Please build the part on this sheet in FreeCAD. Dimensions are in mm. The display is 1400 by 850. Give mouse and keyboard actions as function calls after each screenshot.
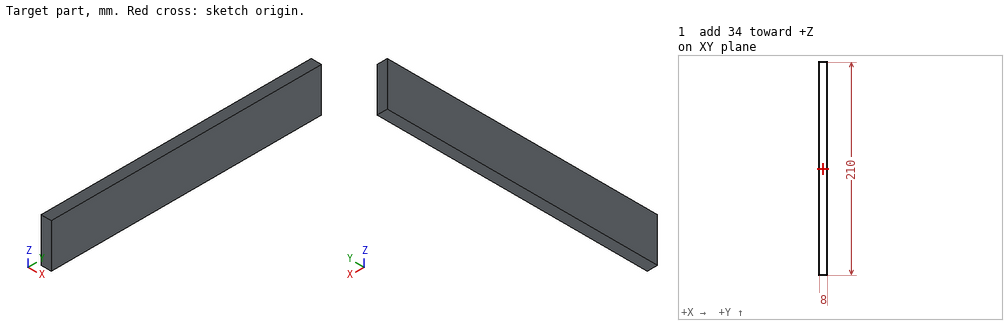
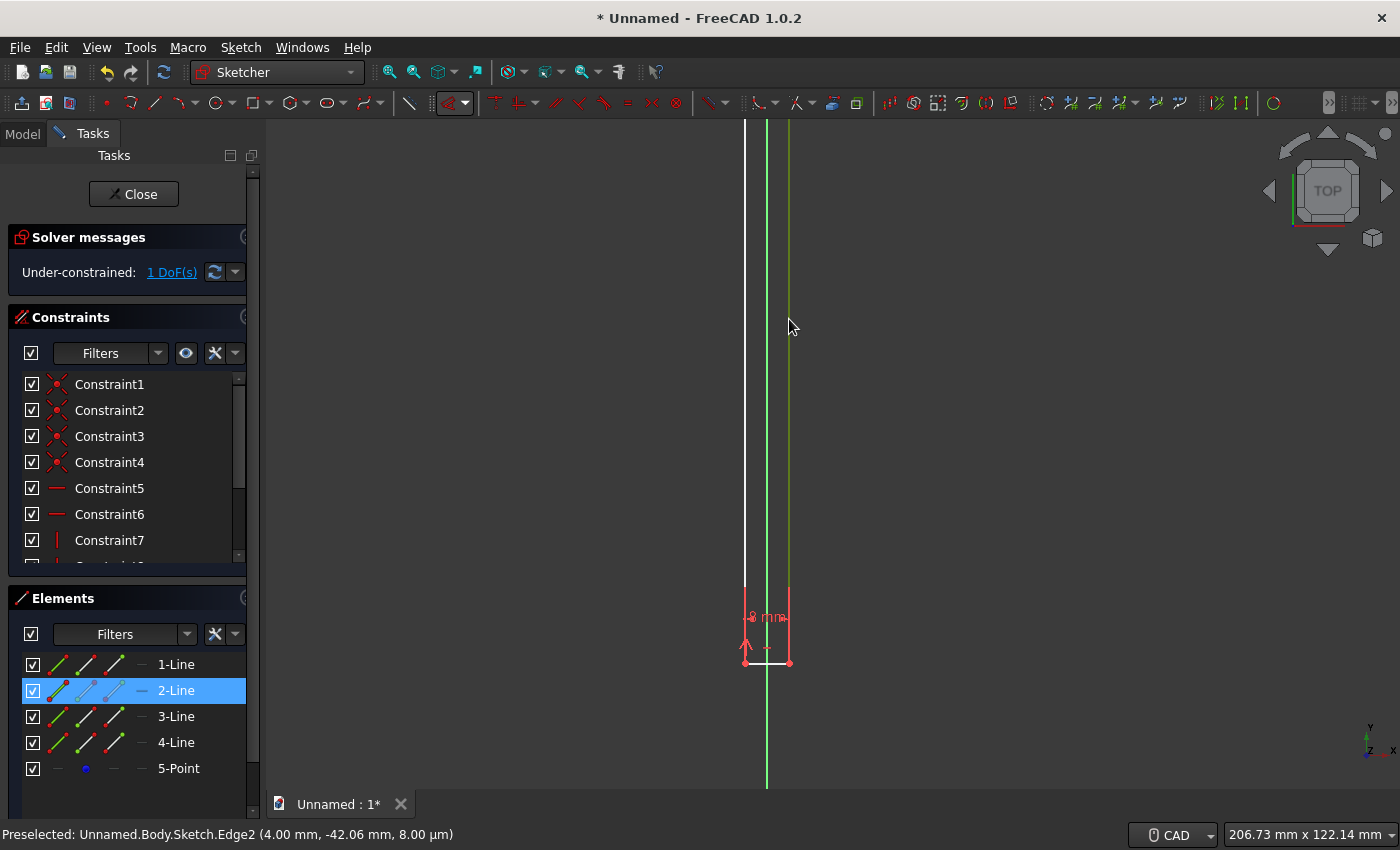
key(i)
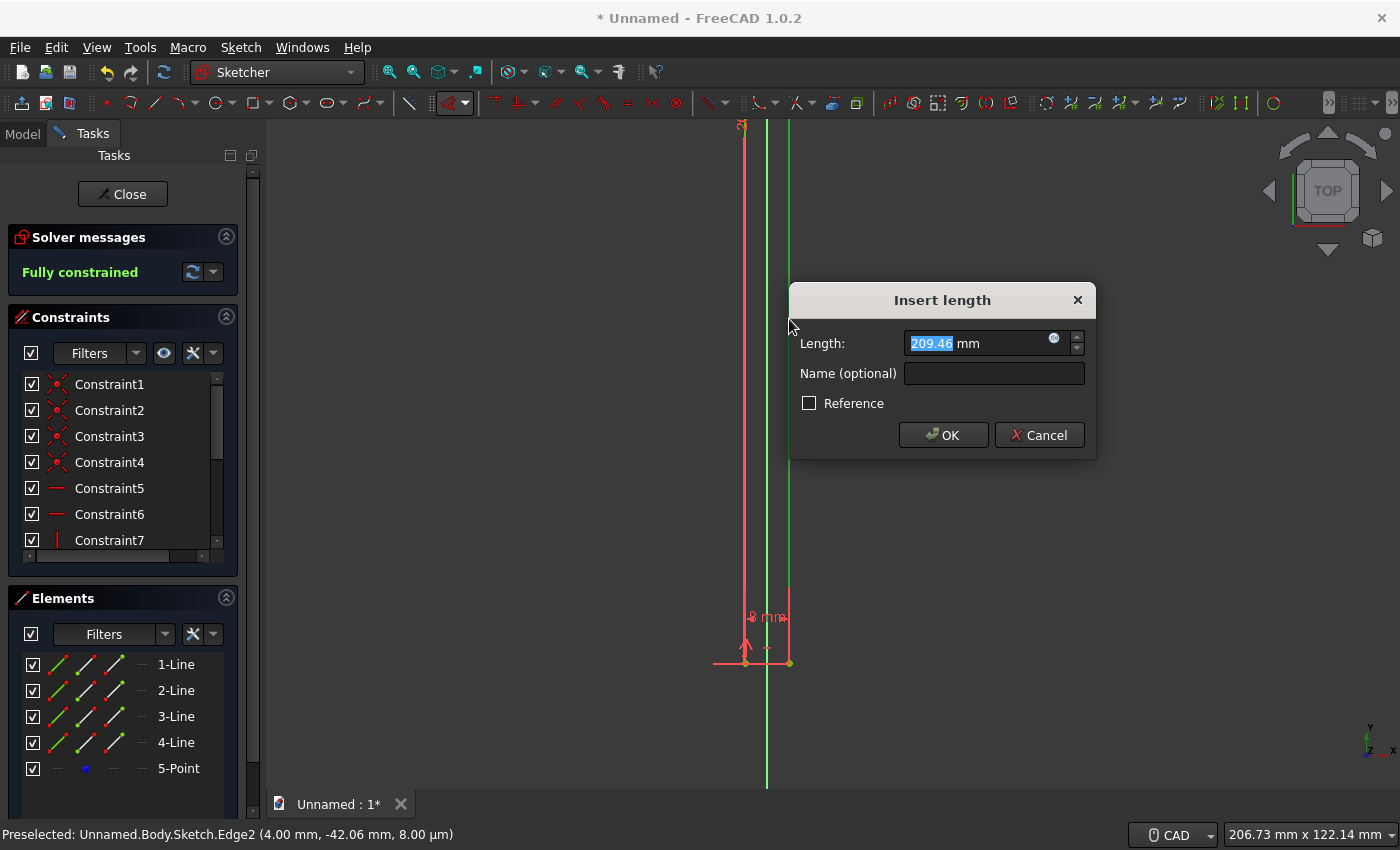
text(210)
key(Return)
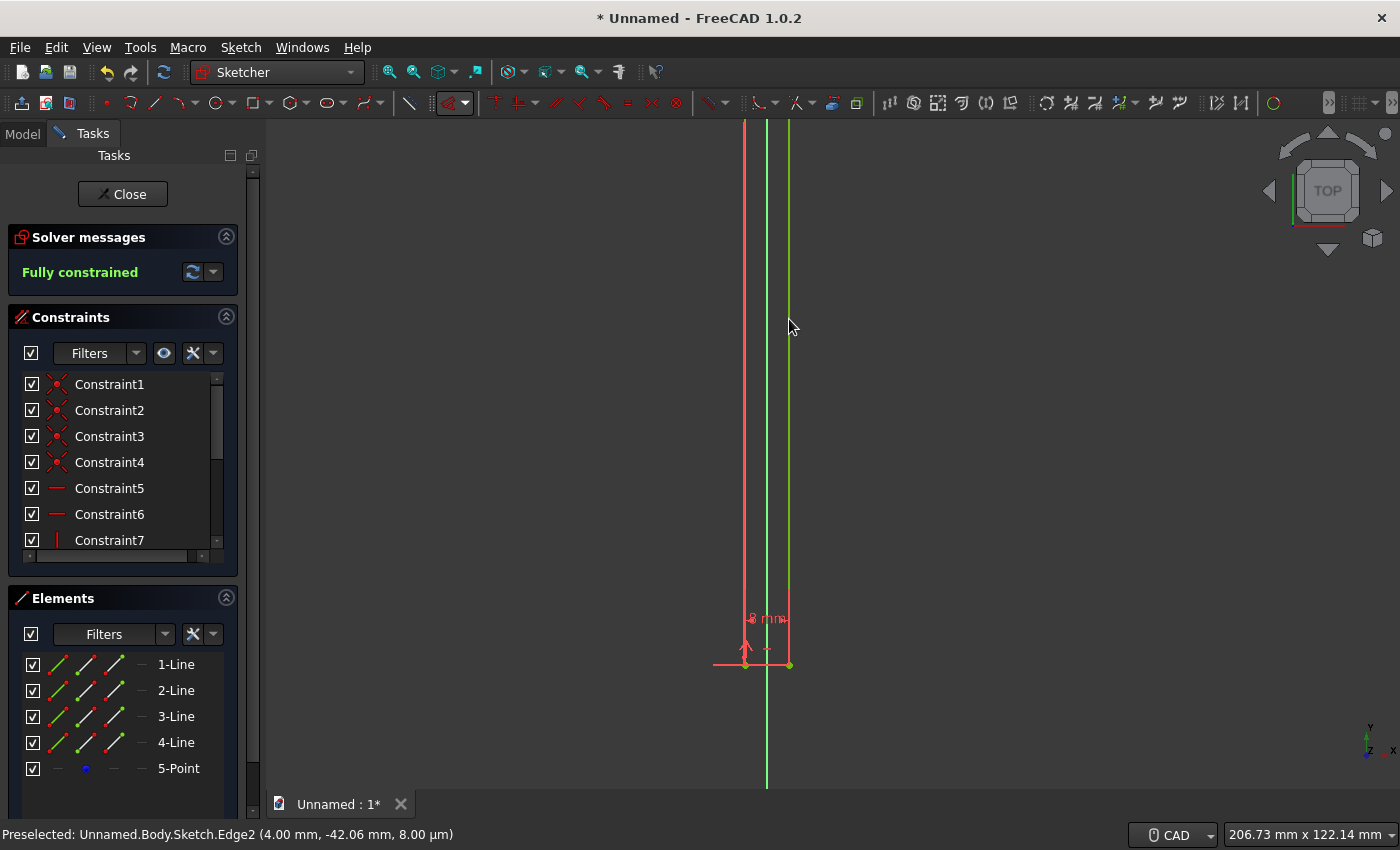
click(123, 194)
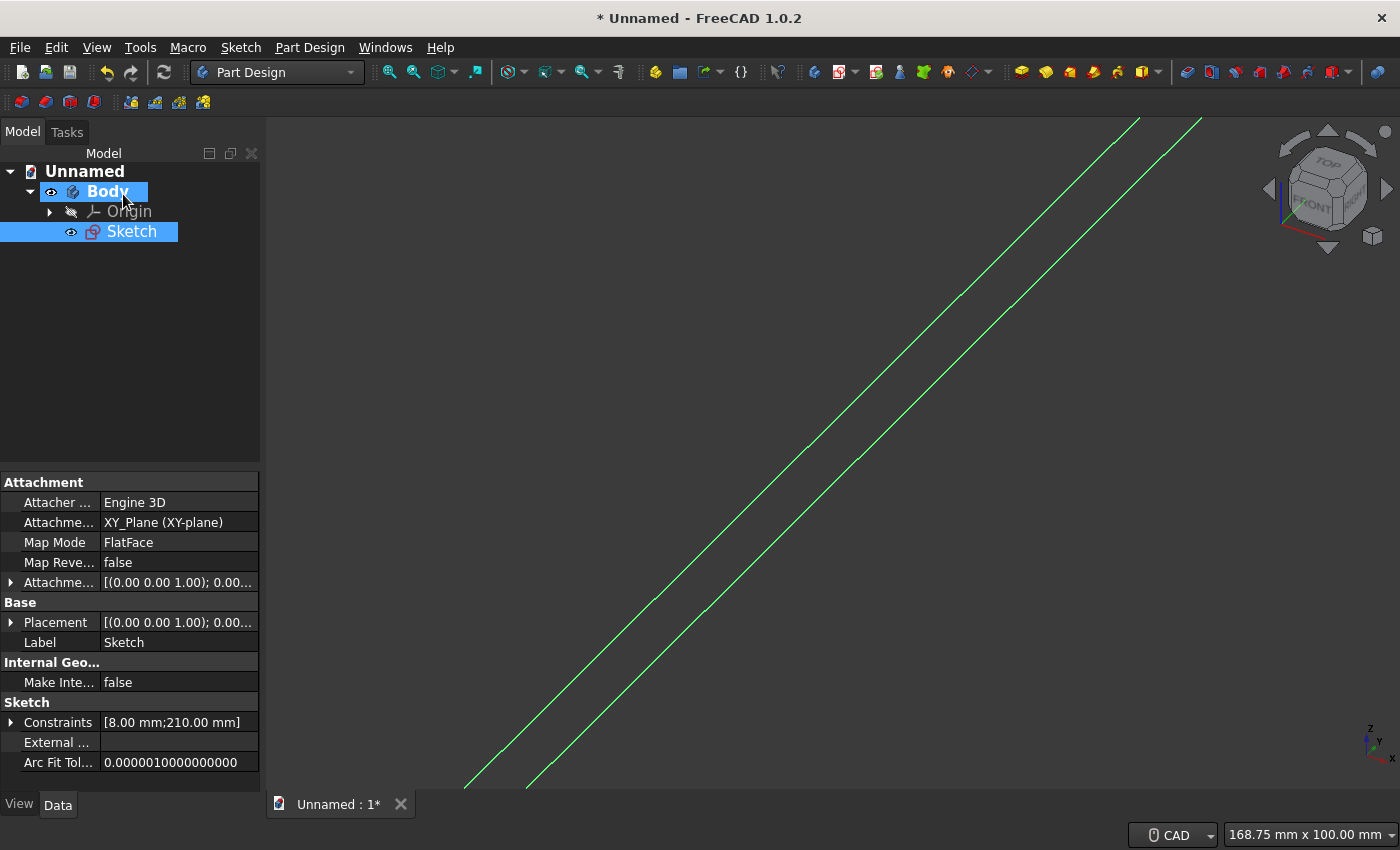
click(1022, 72)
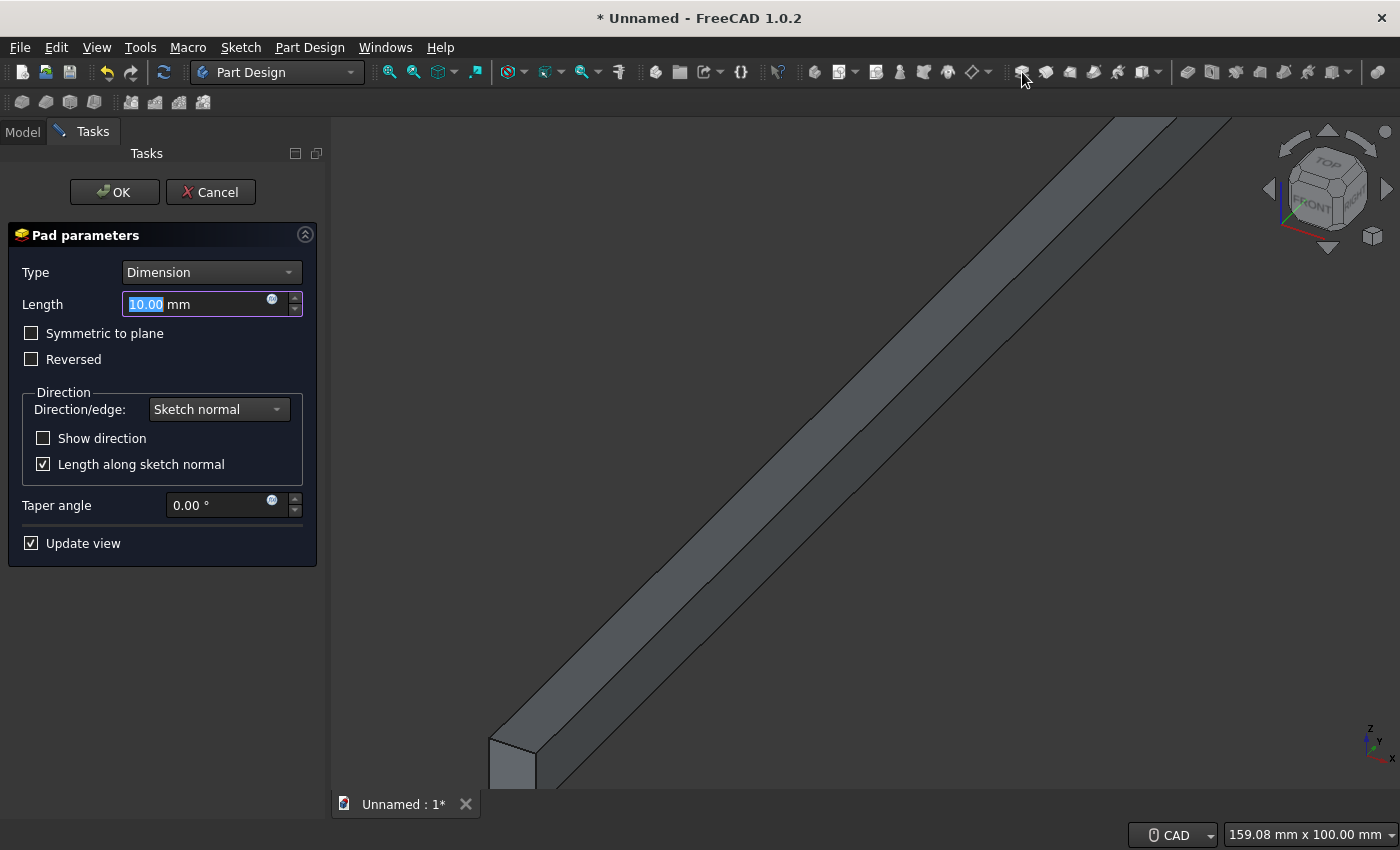
text(34)
key(Tab)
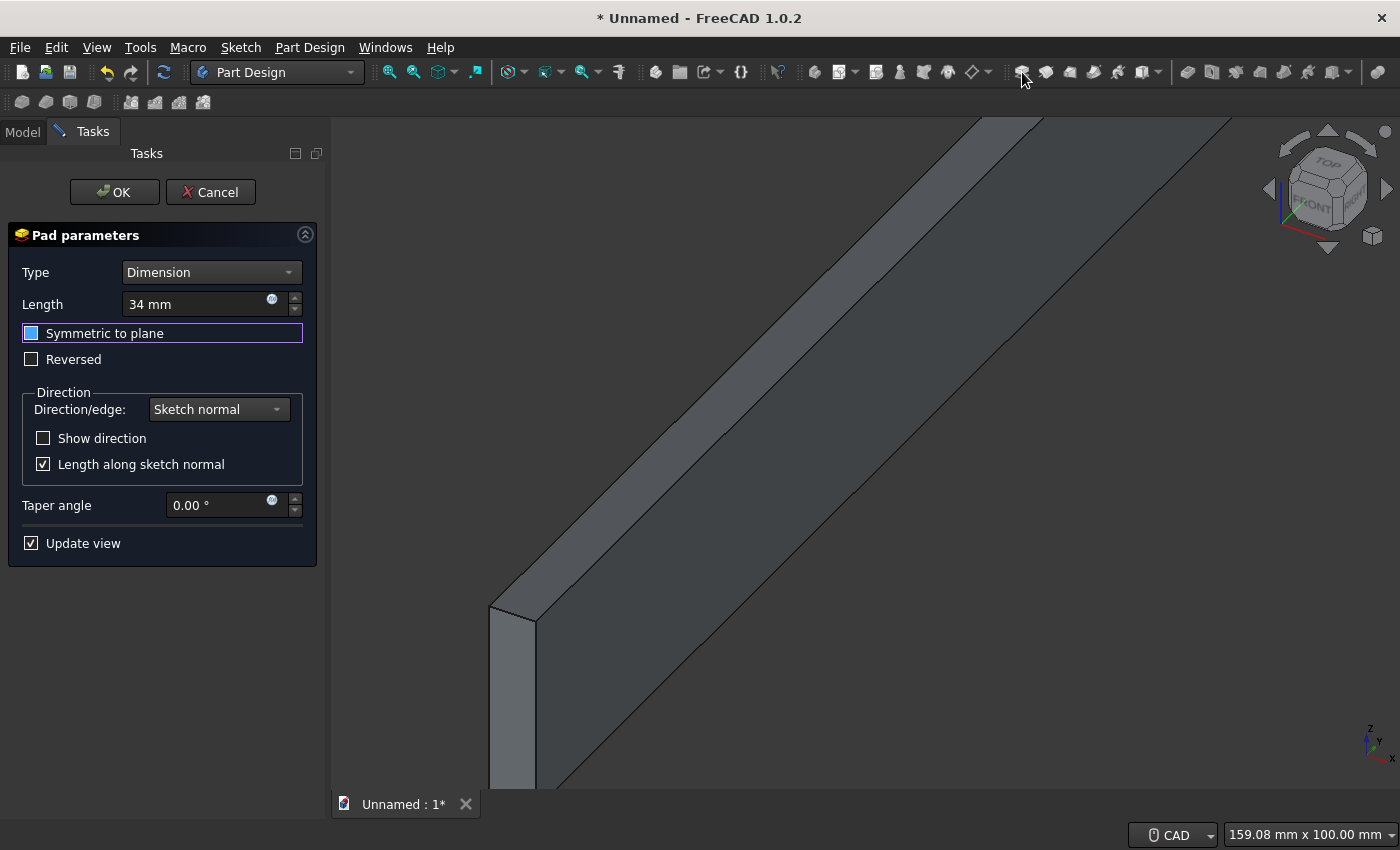
click(115, 192)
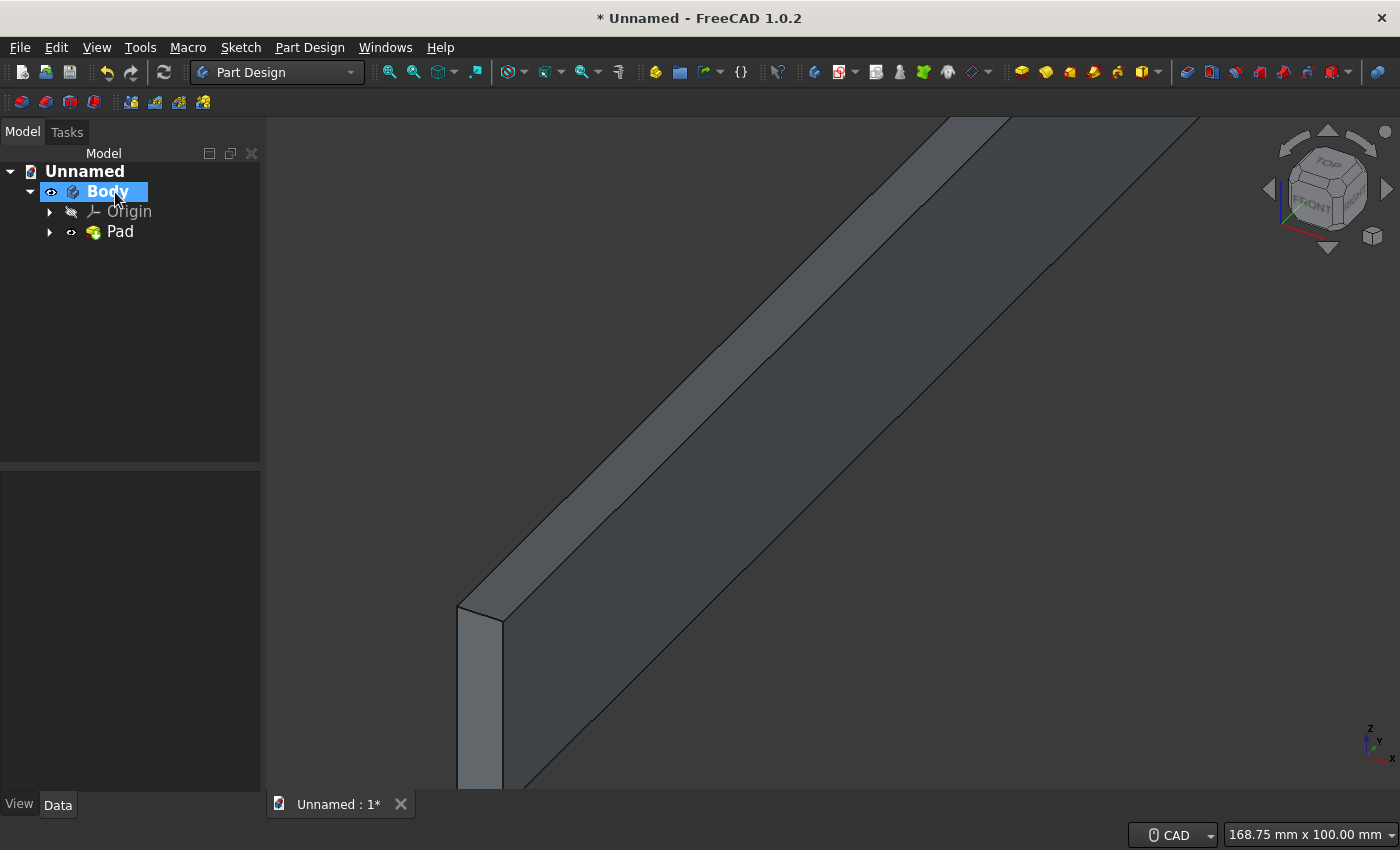
key(0)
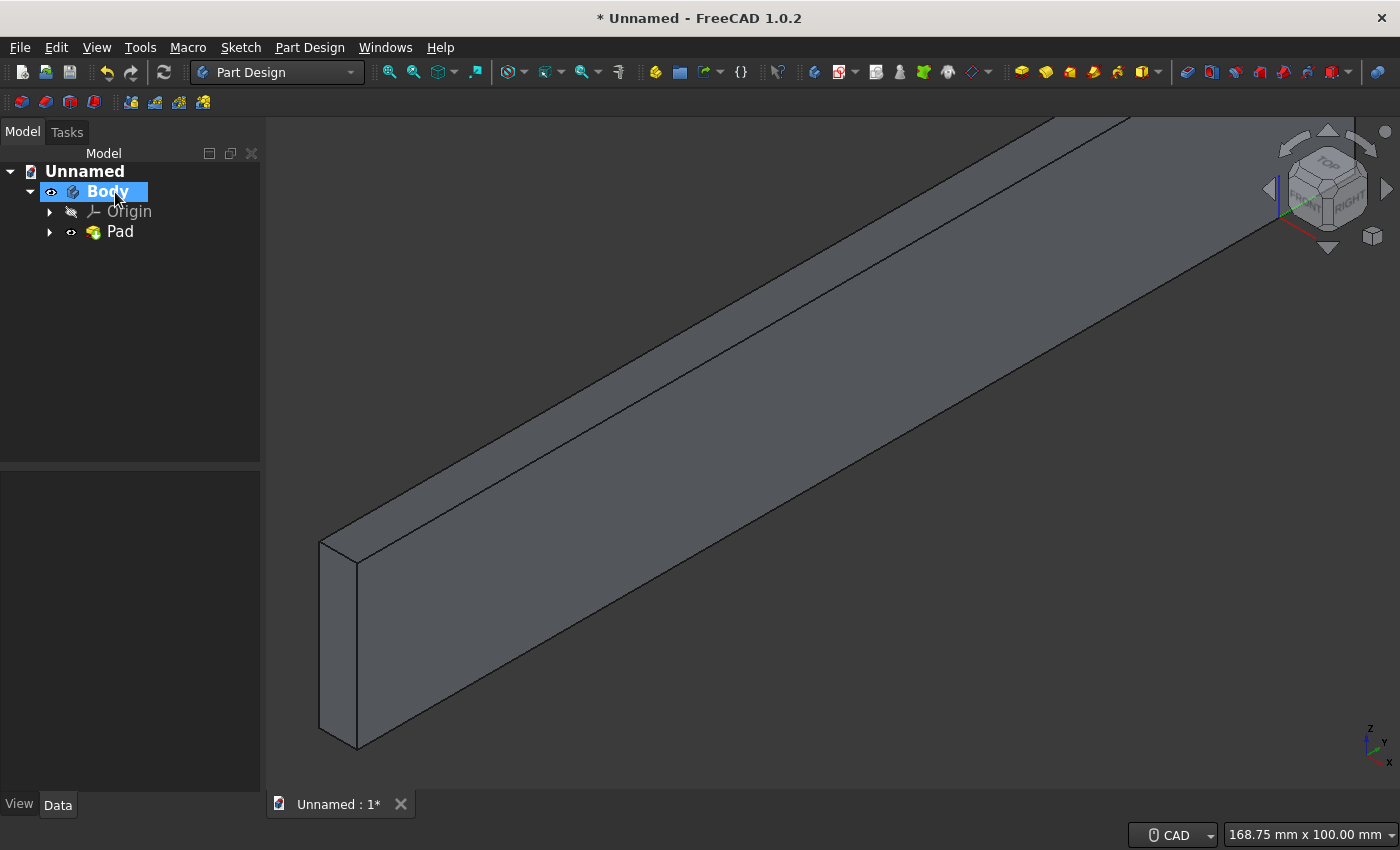
click(390, 72)